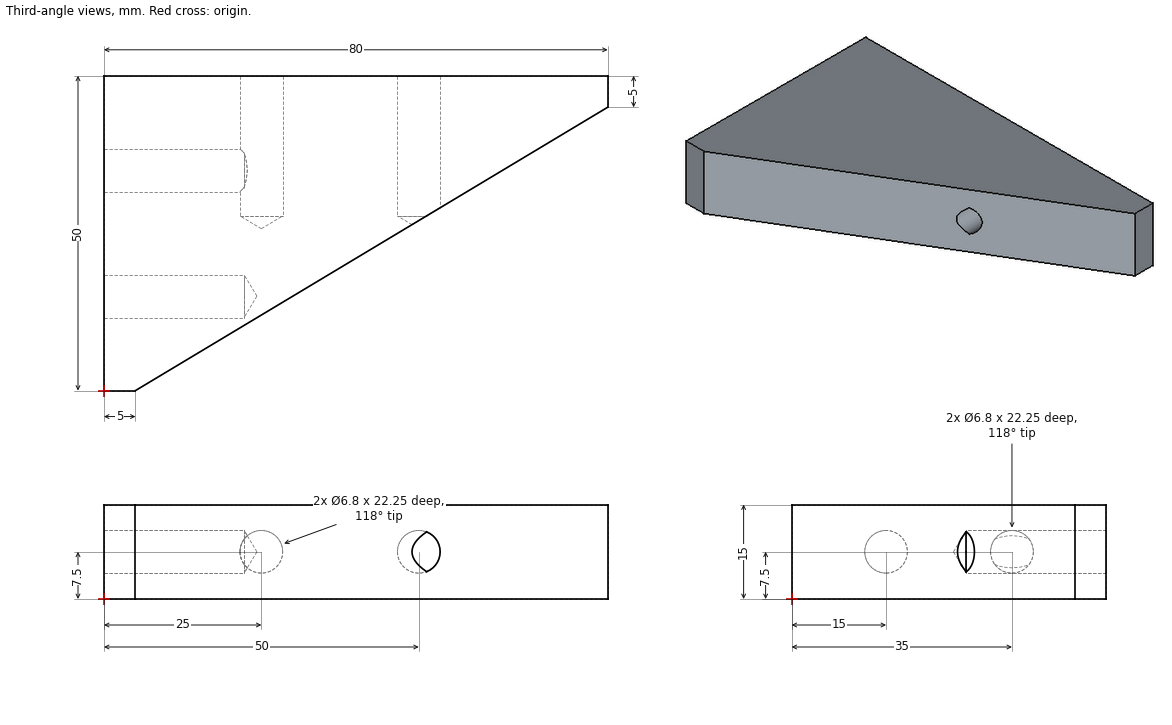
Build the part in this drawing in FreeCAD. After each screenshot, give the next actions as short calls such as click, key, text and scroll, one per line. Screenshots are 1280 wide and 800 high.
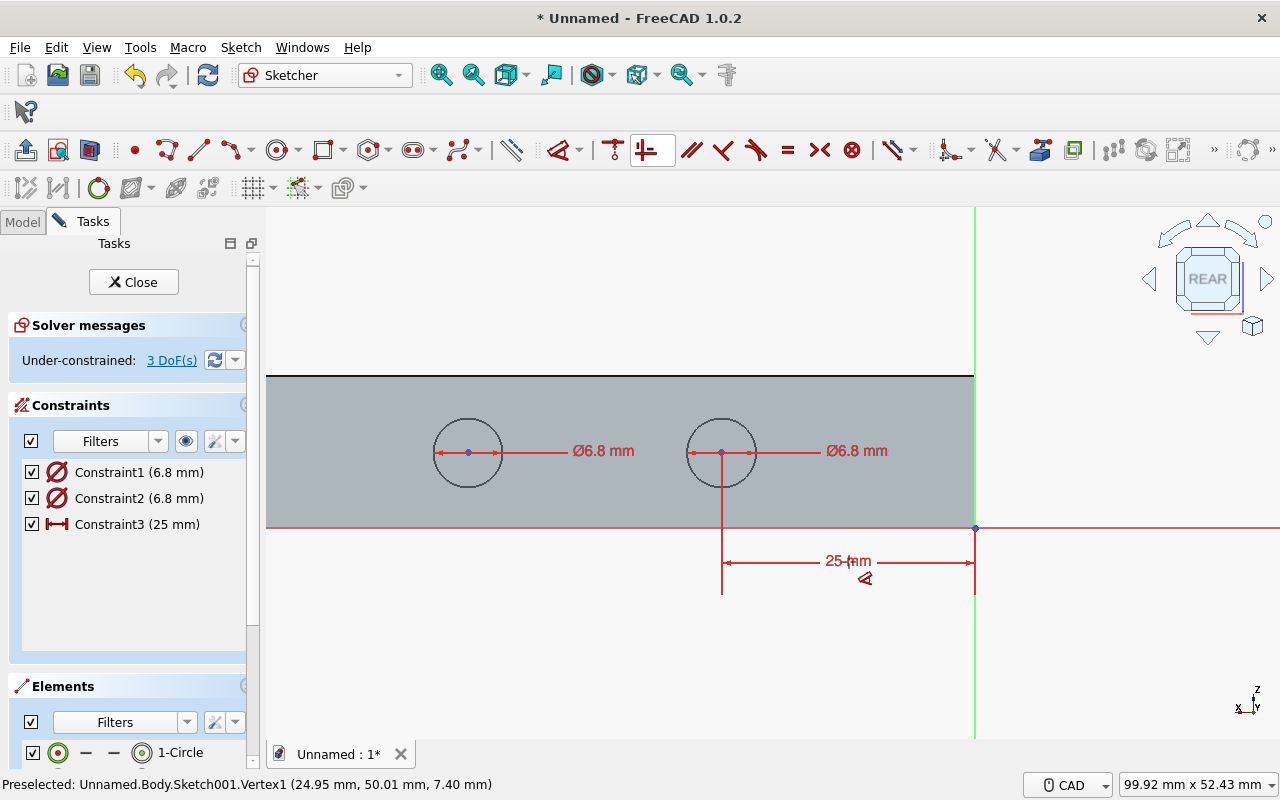
click(468, 453)
click(722, 562)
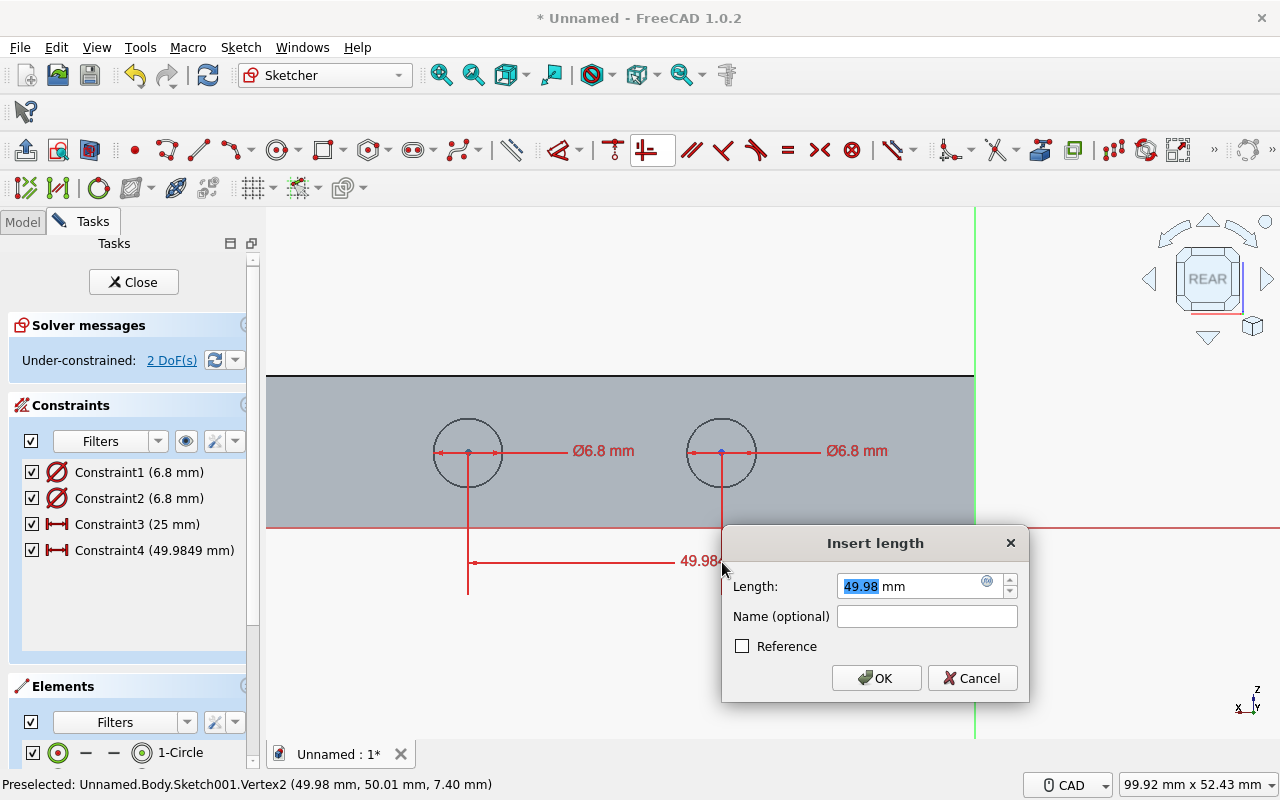
text(50)
key(Return)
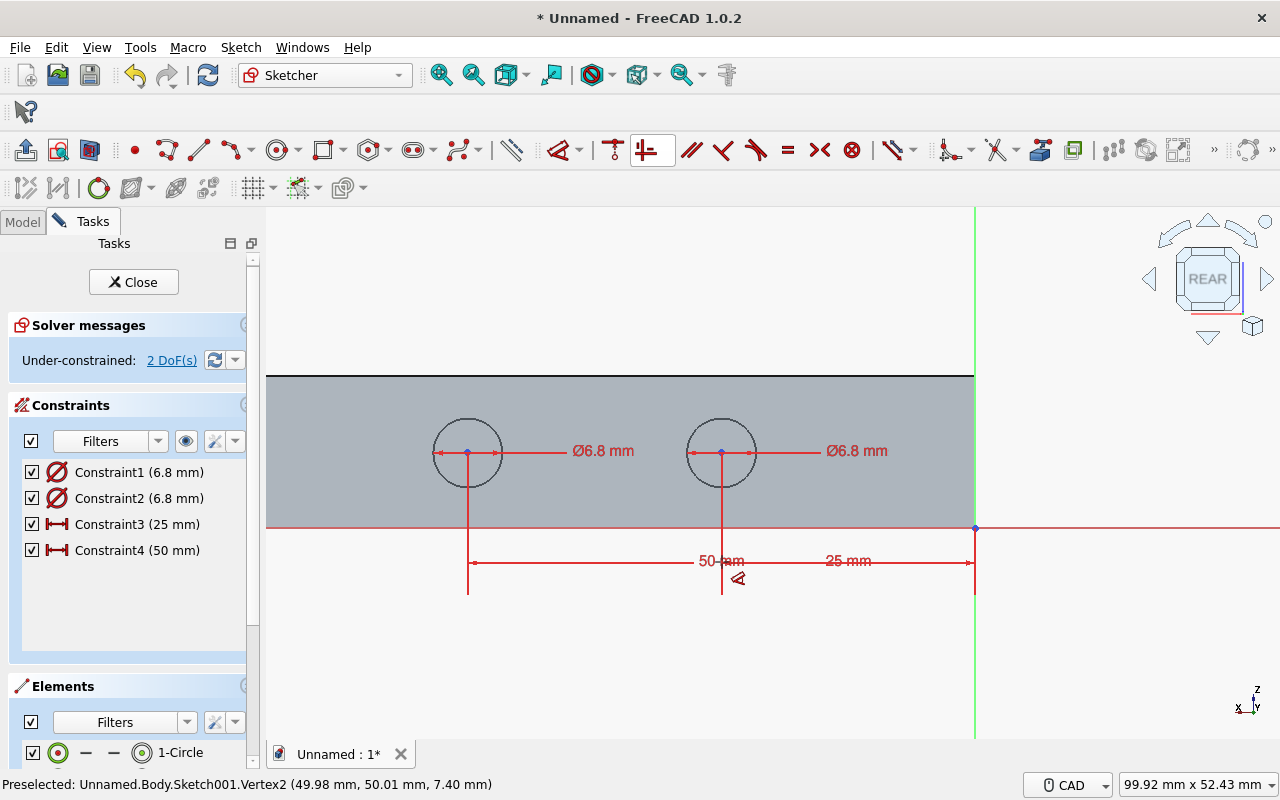
click(722, 453)
click(1009, 491)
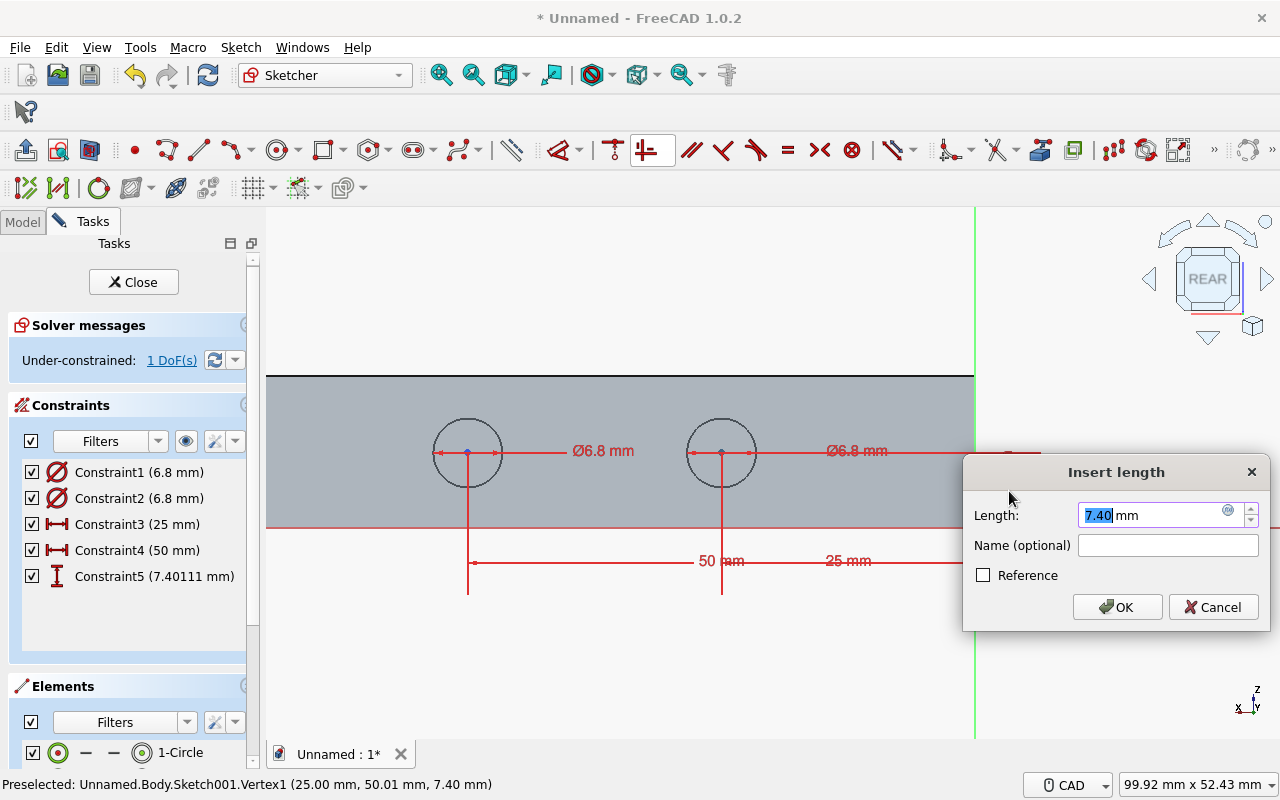
text(7.5)
key(Return)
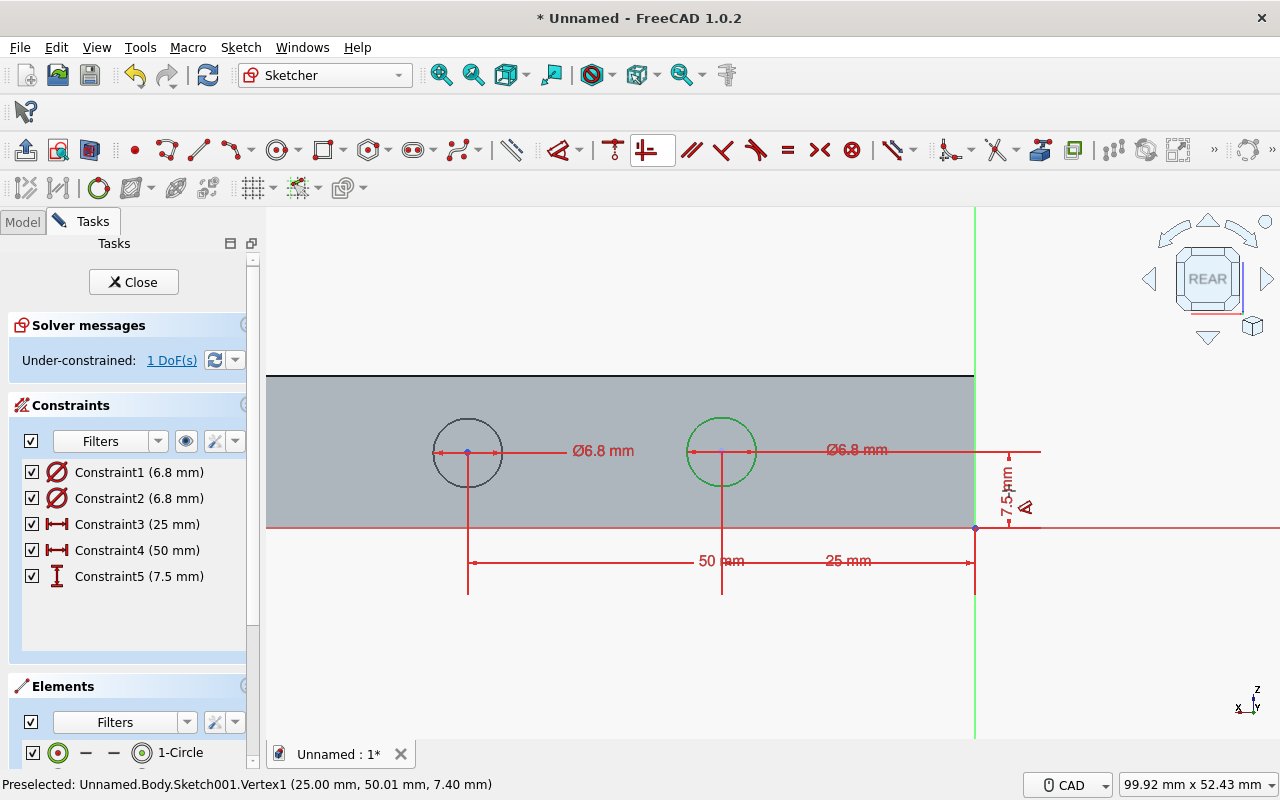
click(468, 453)
click(1009, 464)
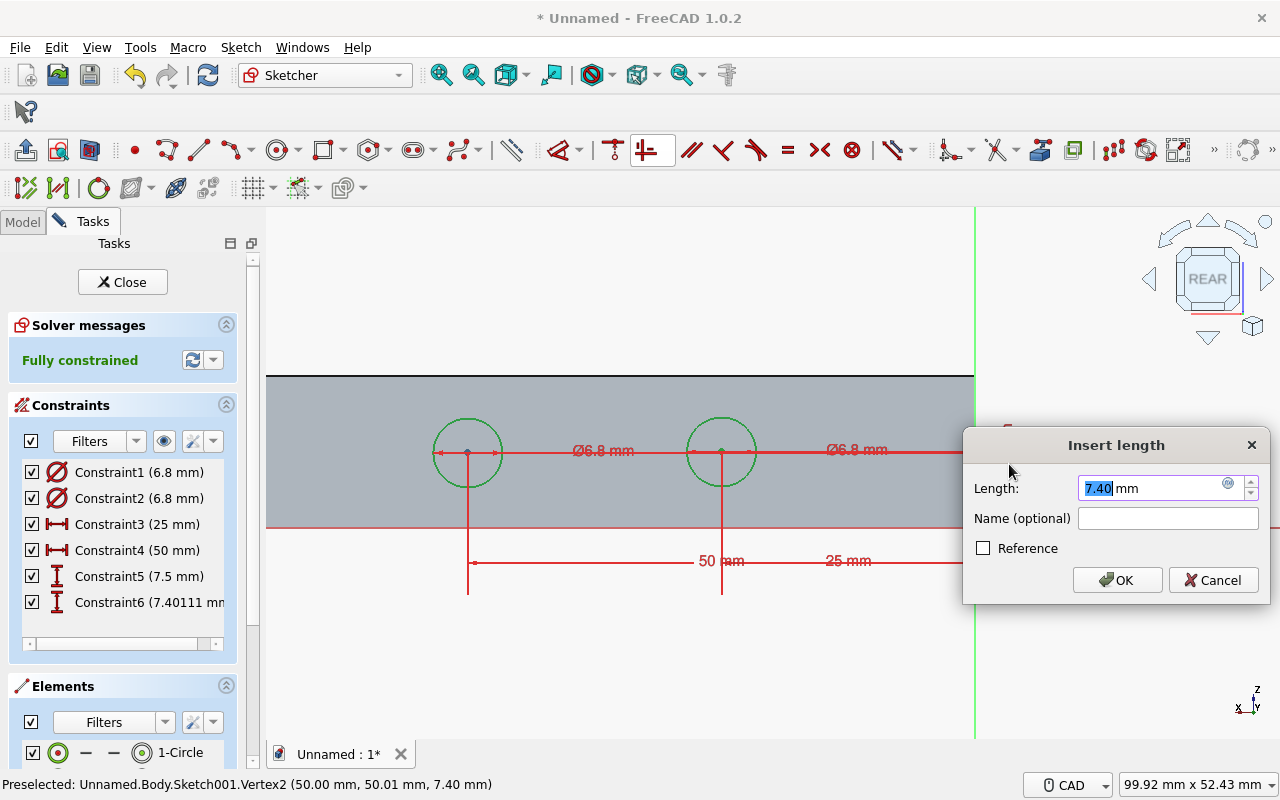
text(7.5)
key(Return)
key(Escape)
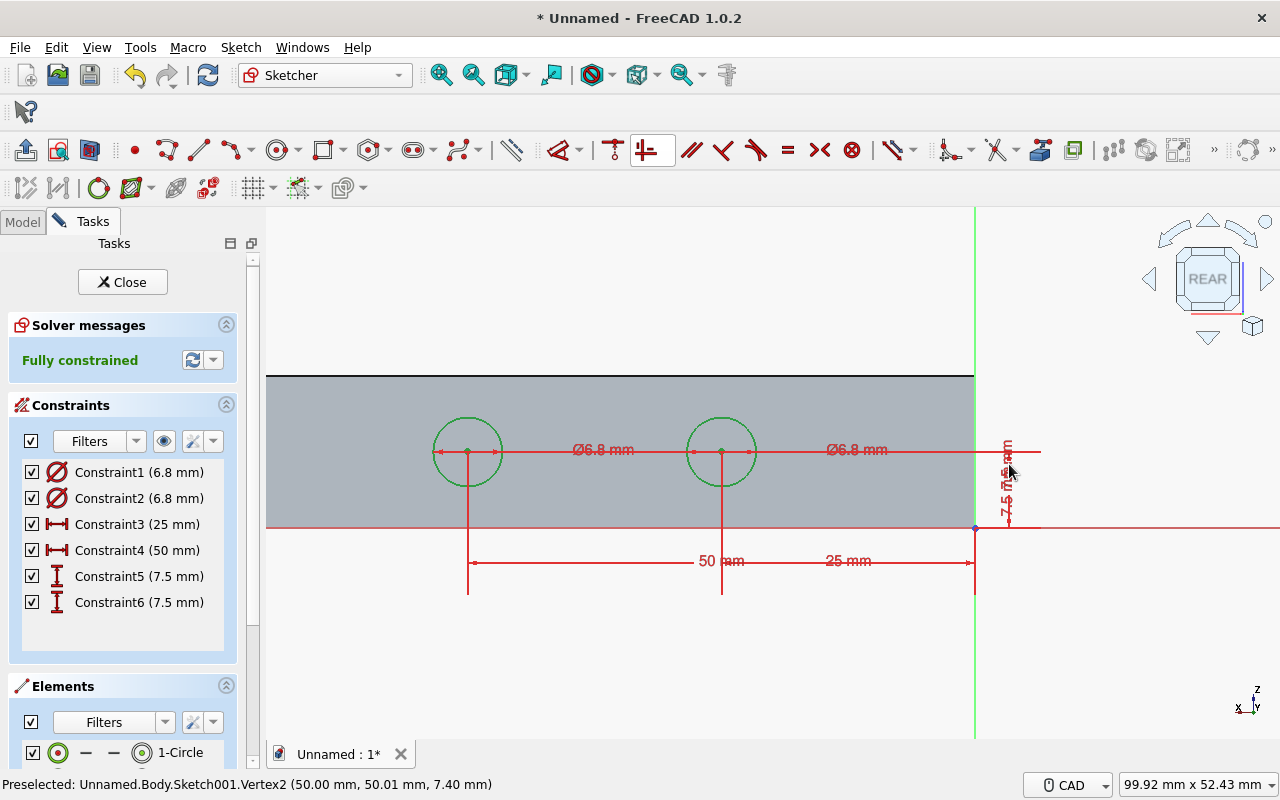
click(123, 282)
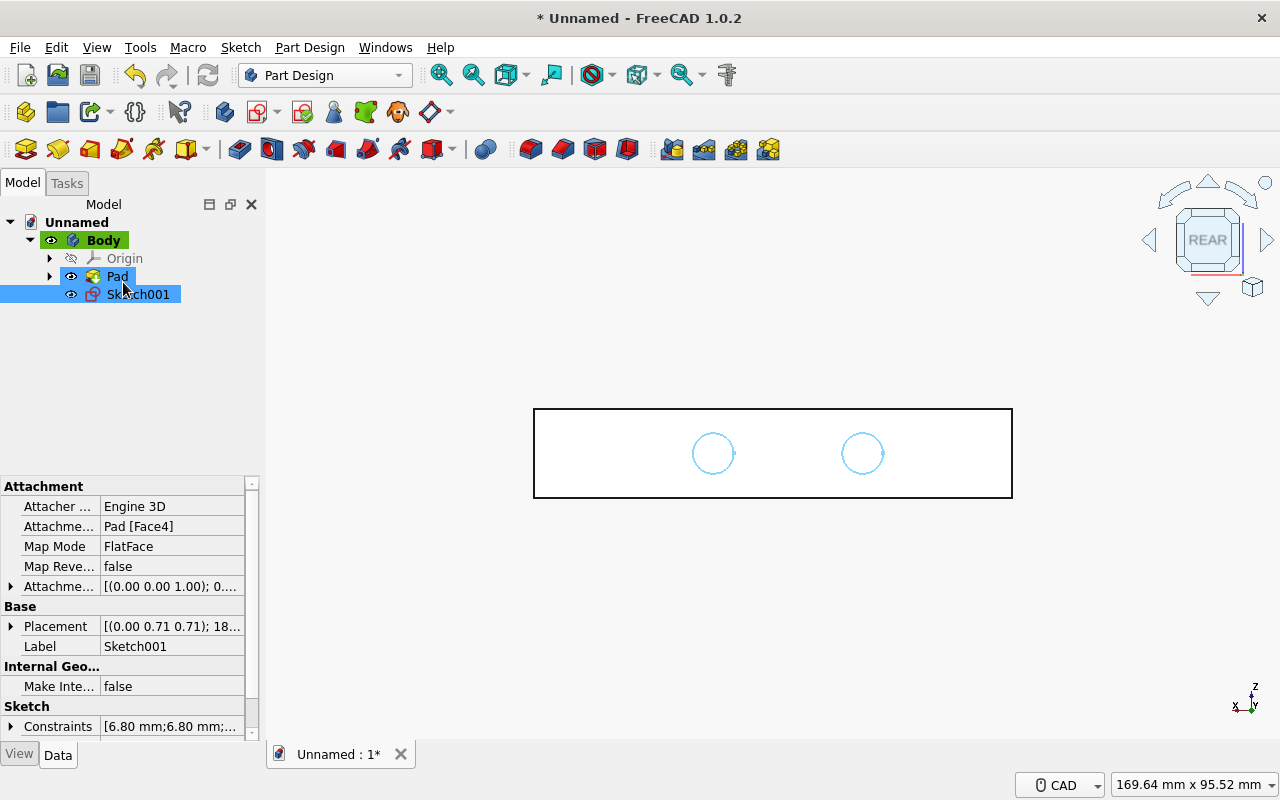
click(272, 150)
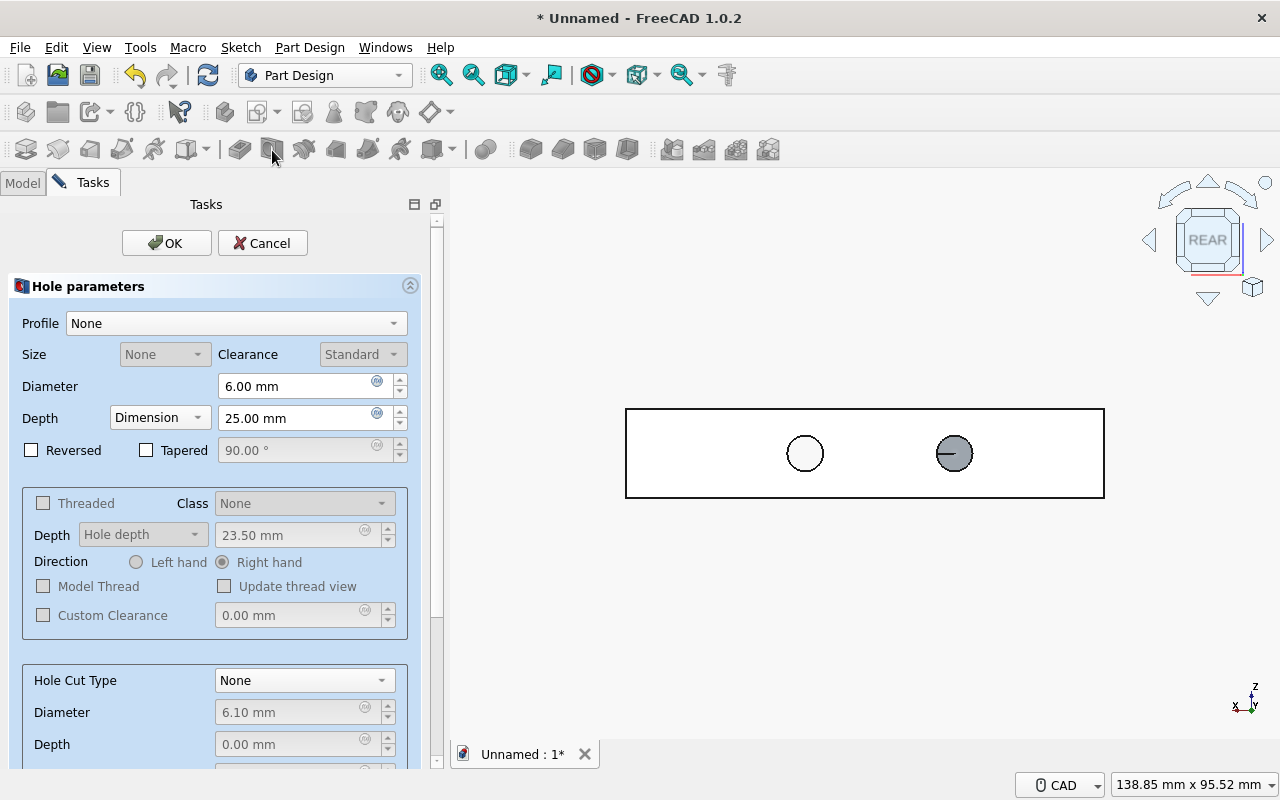
triple_click(305, 386)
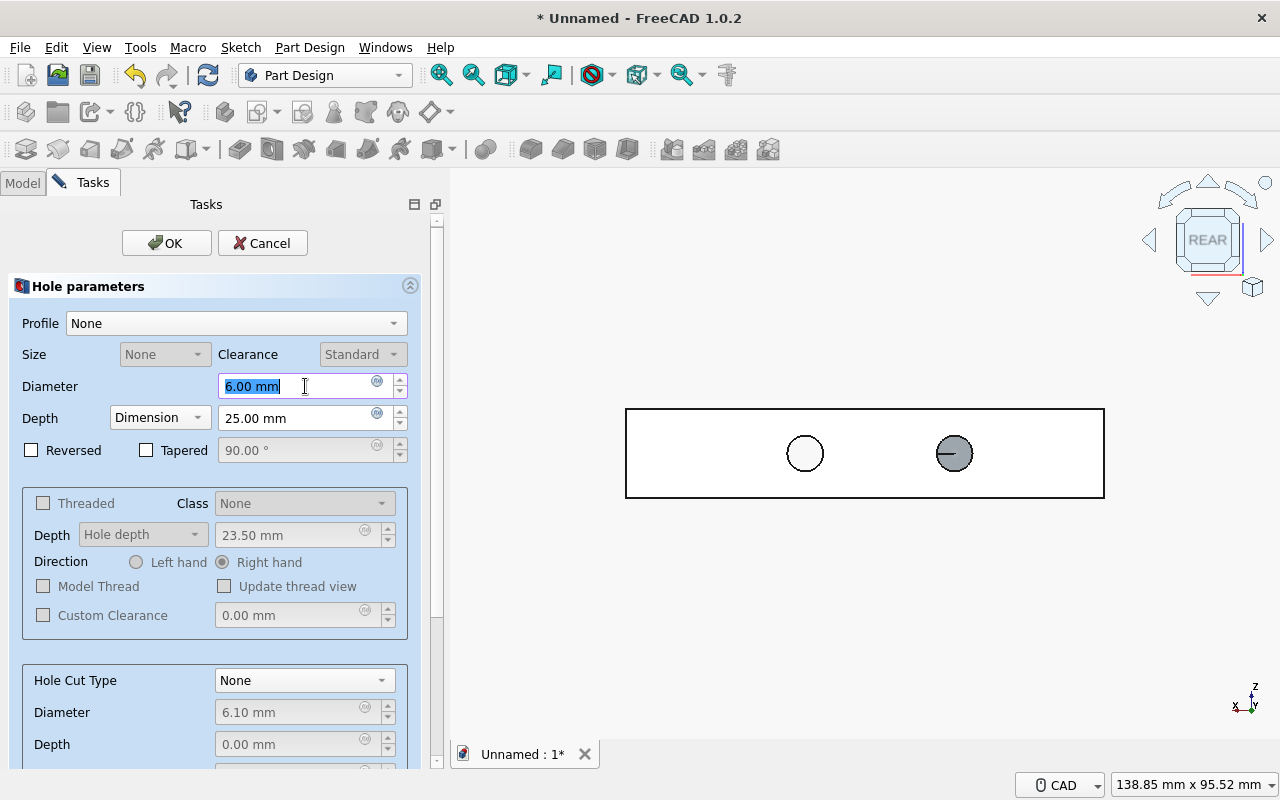
text(6.8)
key(Tab)